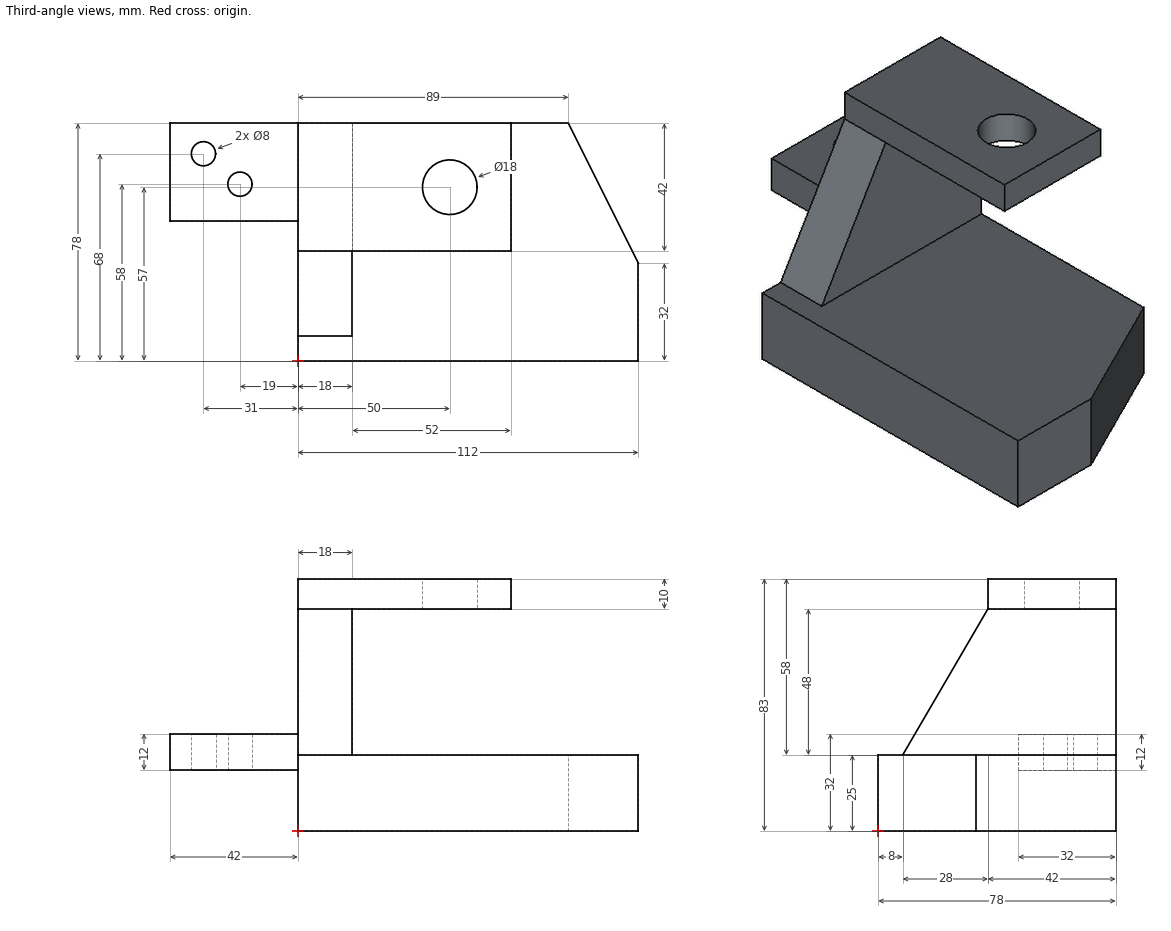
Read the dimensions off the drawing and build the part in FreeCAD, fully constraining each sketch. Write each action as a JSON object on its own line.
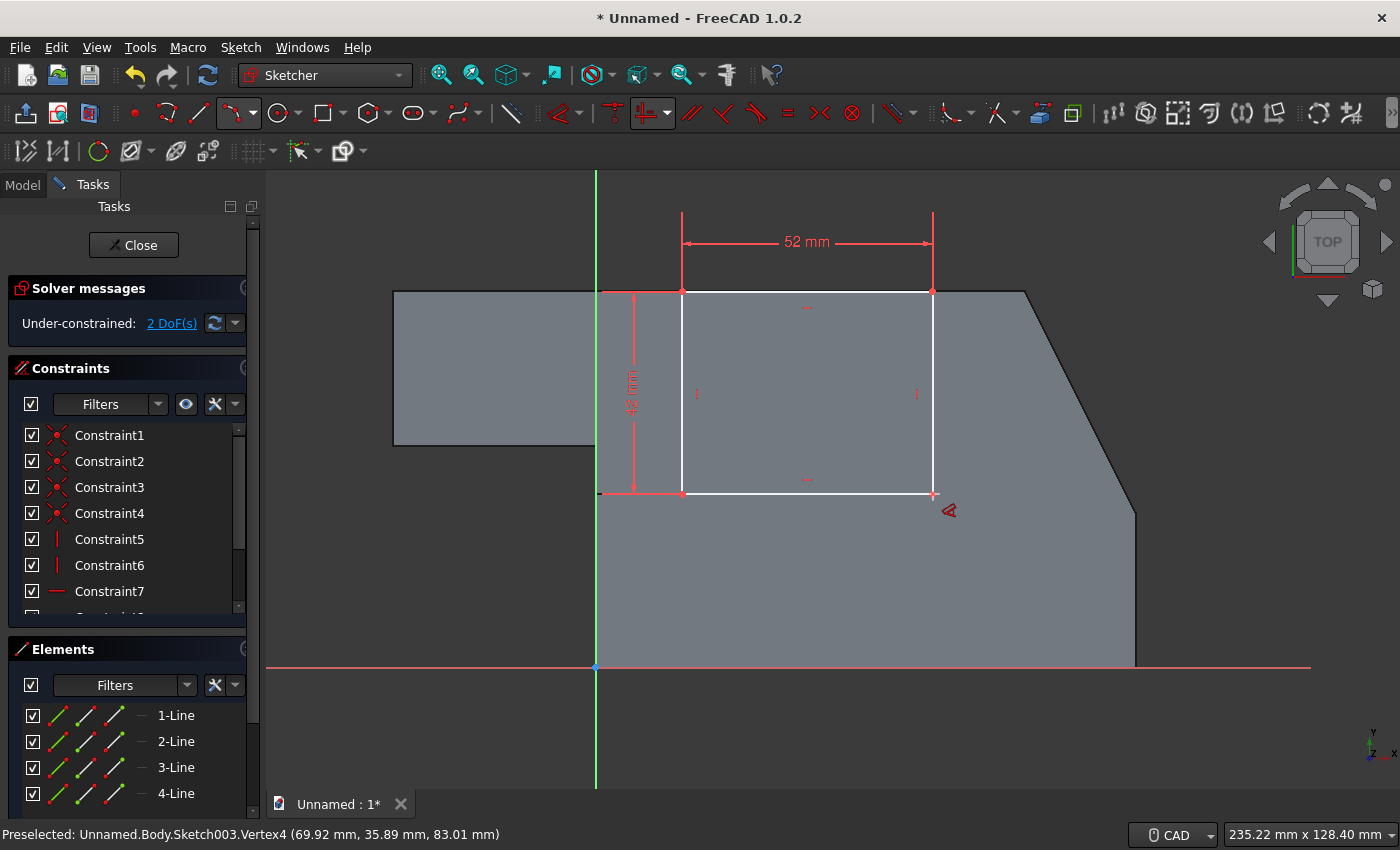
{"action": "left_click", "coordinate": [682, 292]}
{"action": "left_click", "coordinate": [639, 702]}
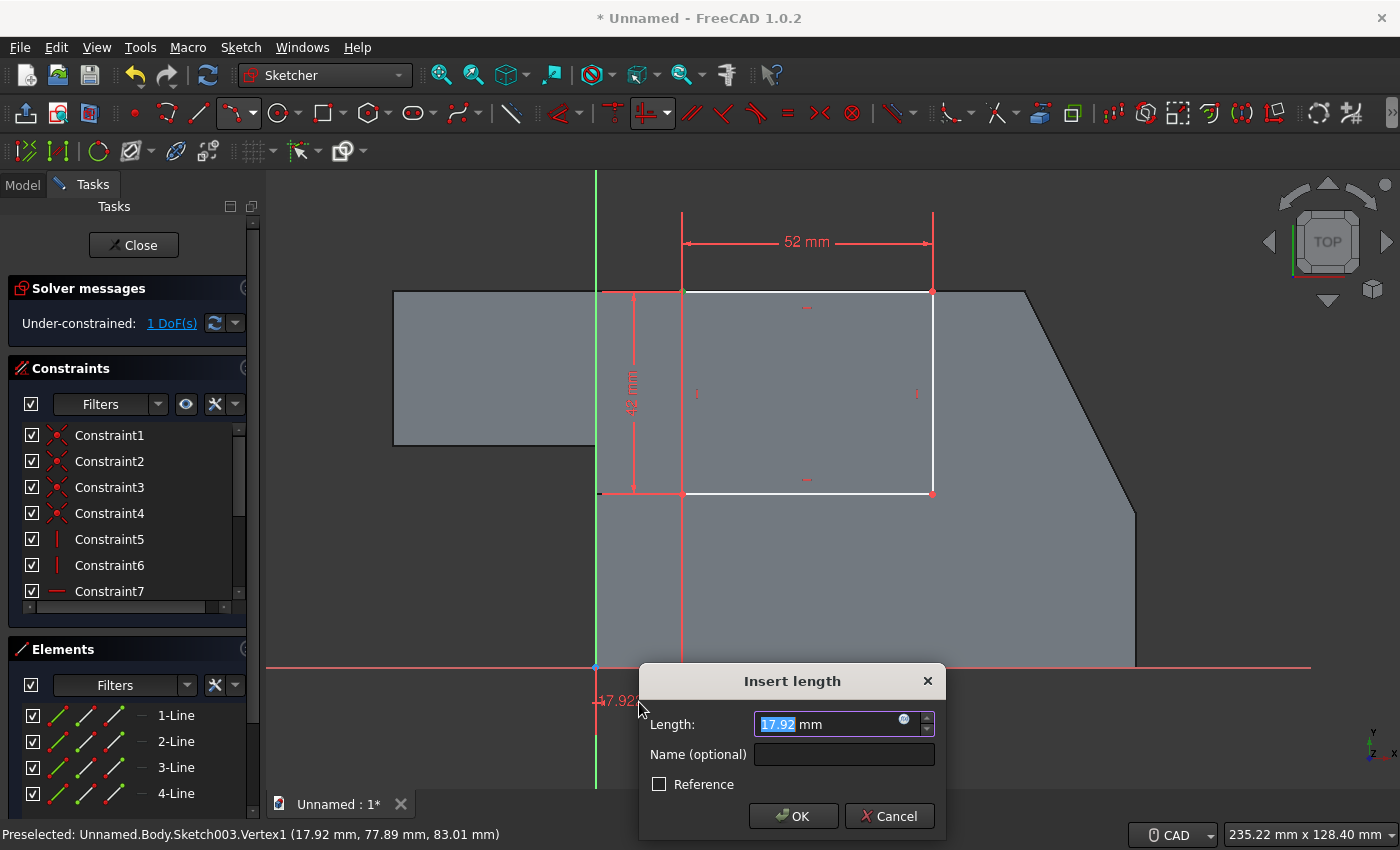
{"action": "type", "text": "18"}
{"action": "key", "text": "Return"}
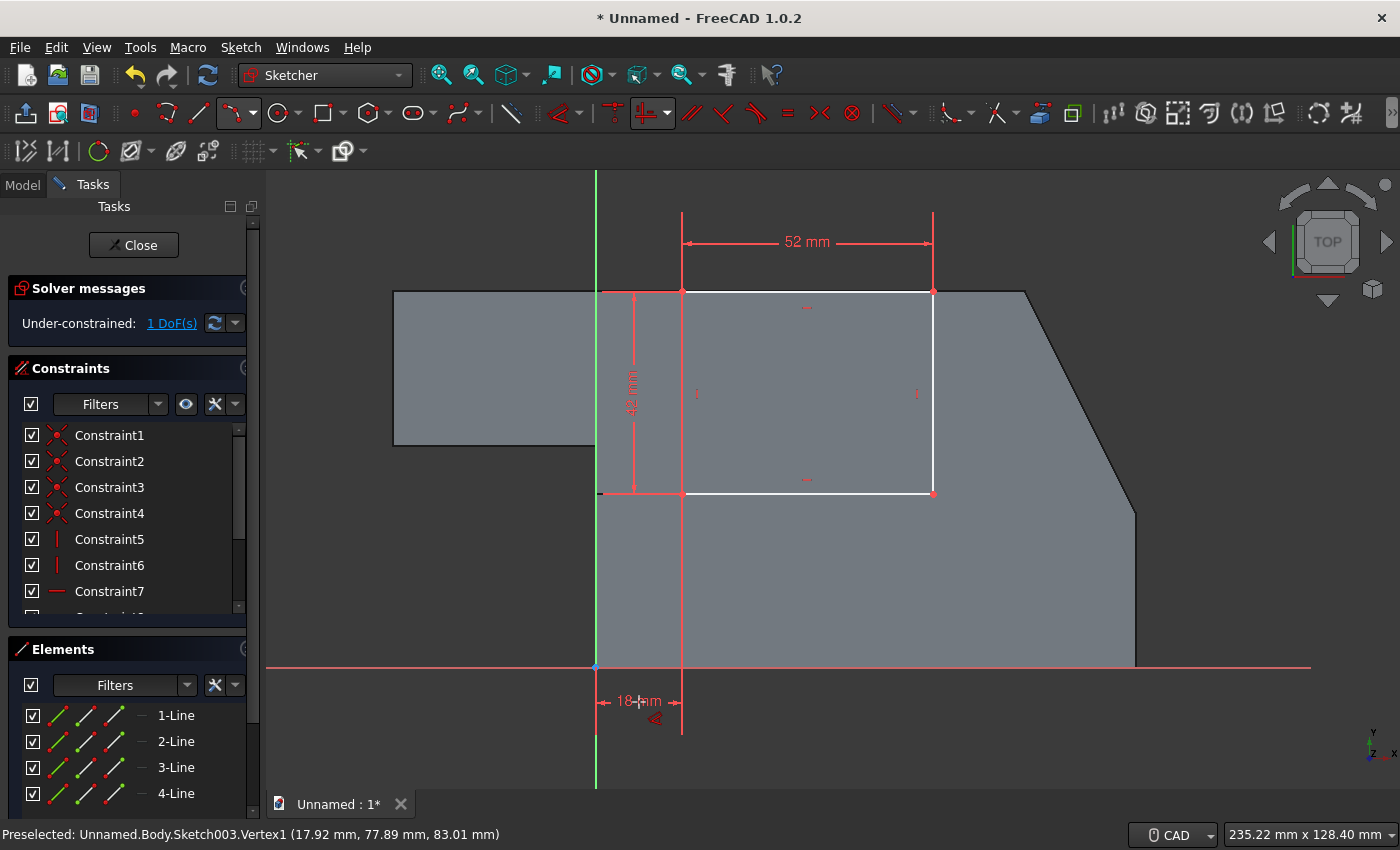
{"action": "left_click", "coordinate": [682, 292]}
{"action": "left_click", "coordinate": [562, 480]}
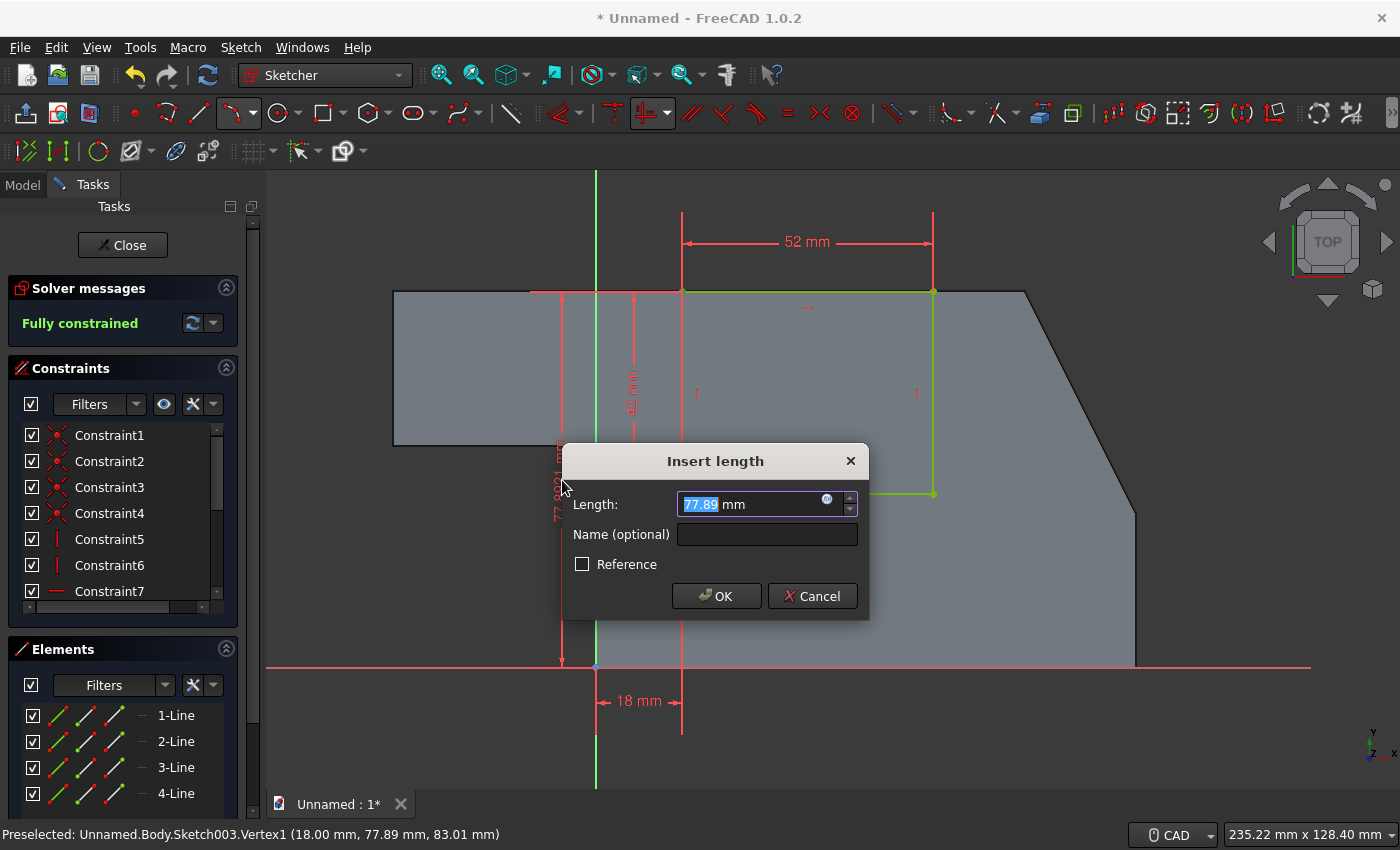
{"action": "type", "text": "78"}
{"action": "key", "text": "Return"}
{"action": "key", "text": "Escape"}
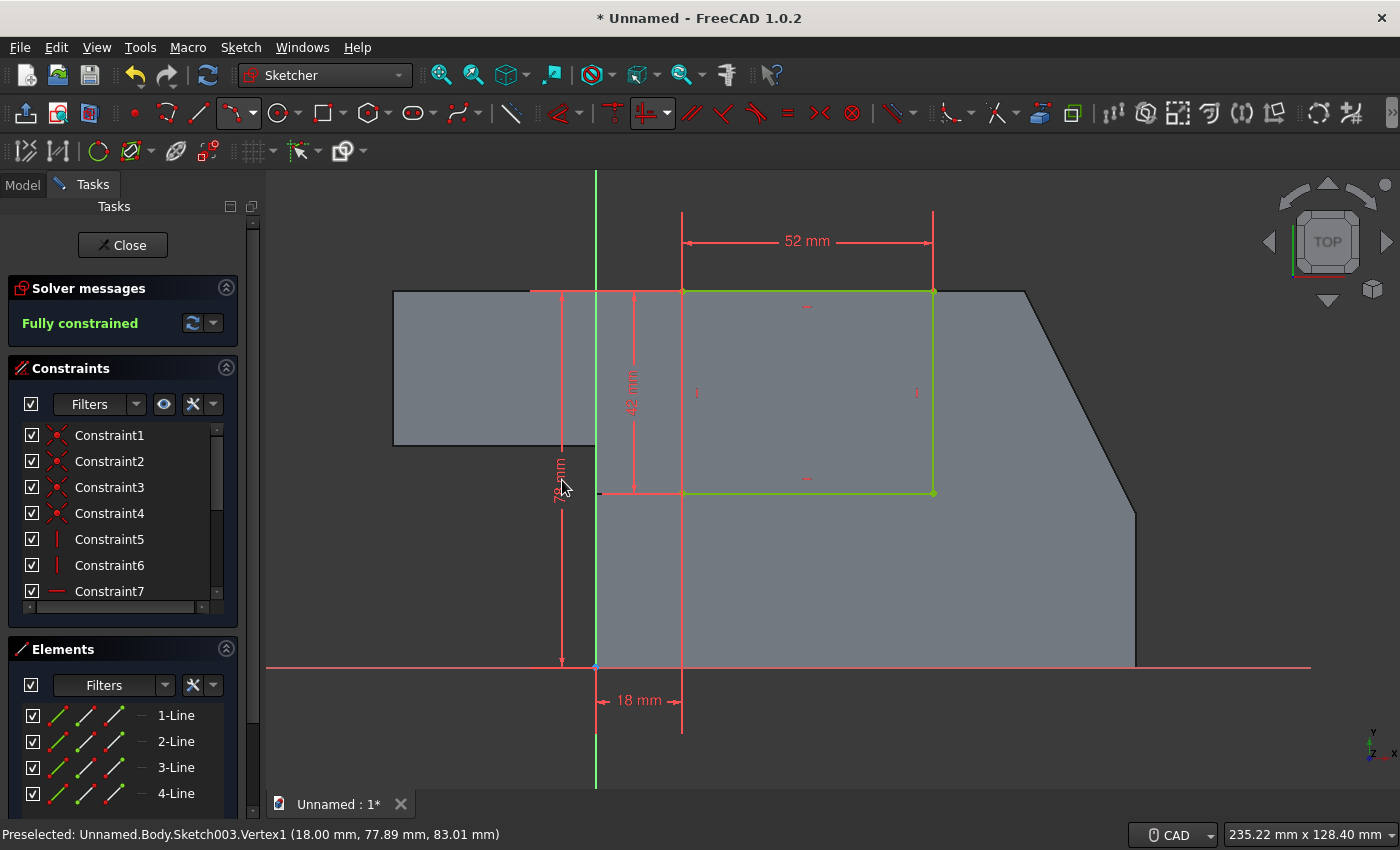
{"action": "left_click", "coordinate": [123, 245]}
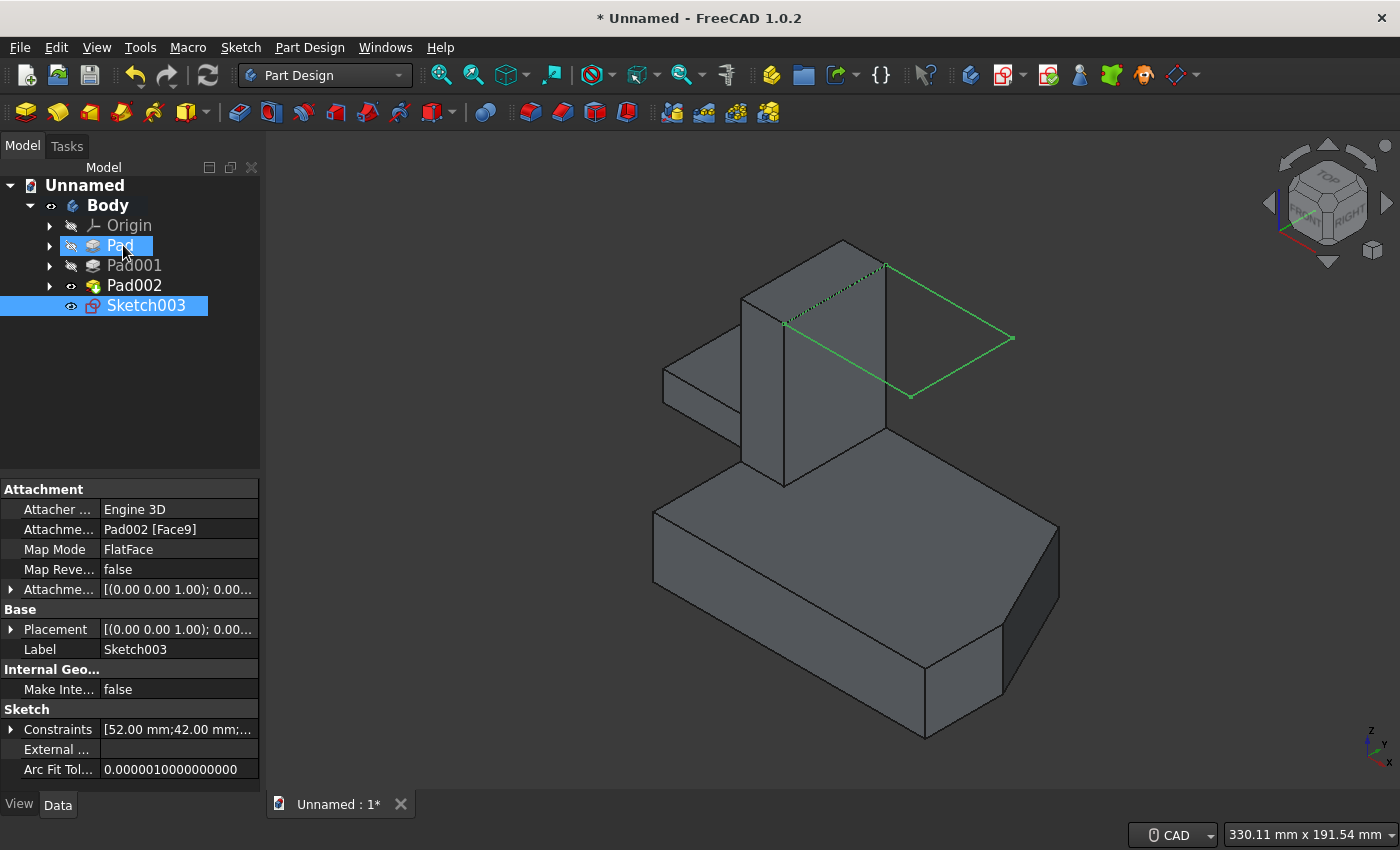
{"action": "left_click", "coordinate": [26, 112]}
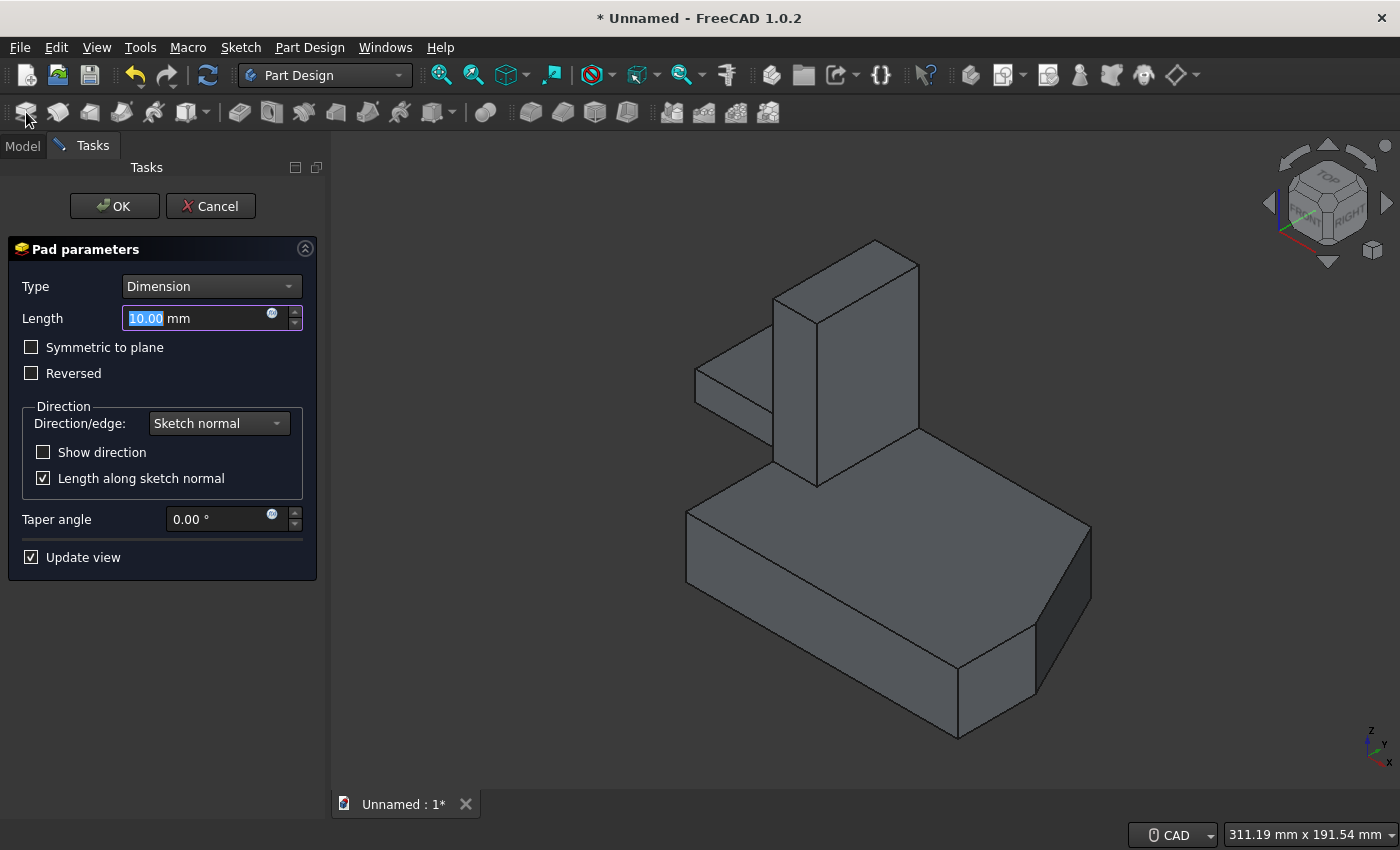
{"action": "type", "text": "10"}
{"action": "key", "text": "Tab"}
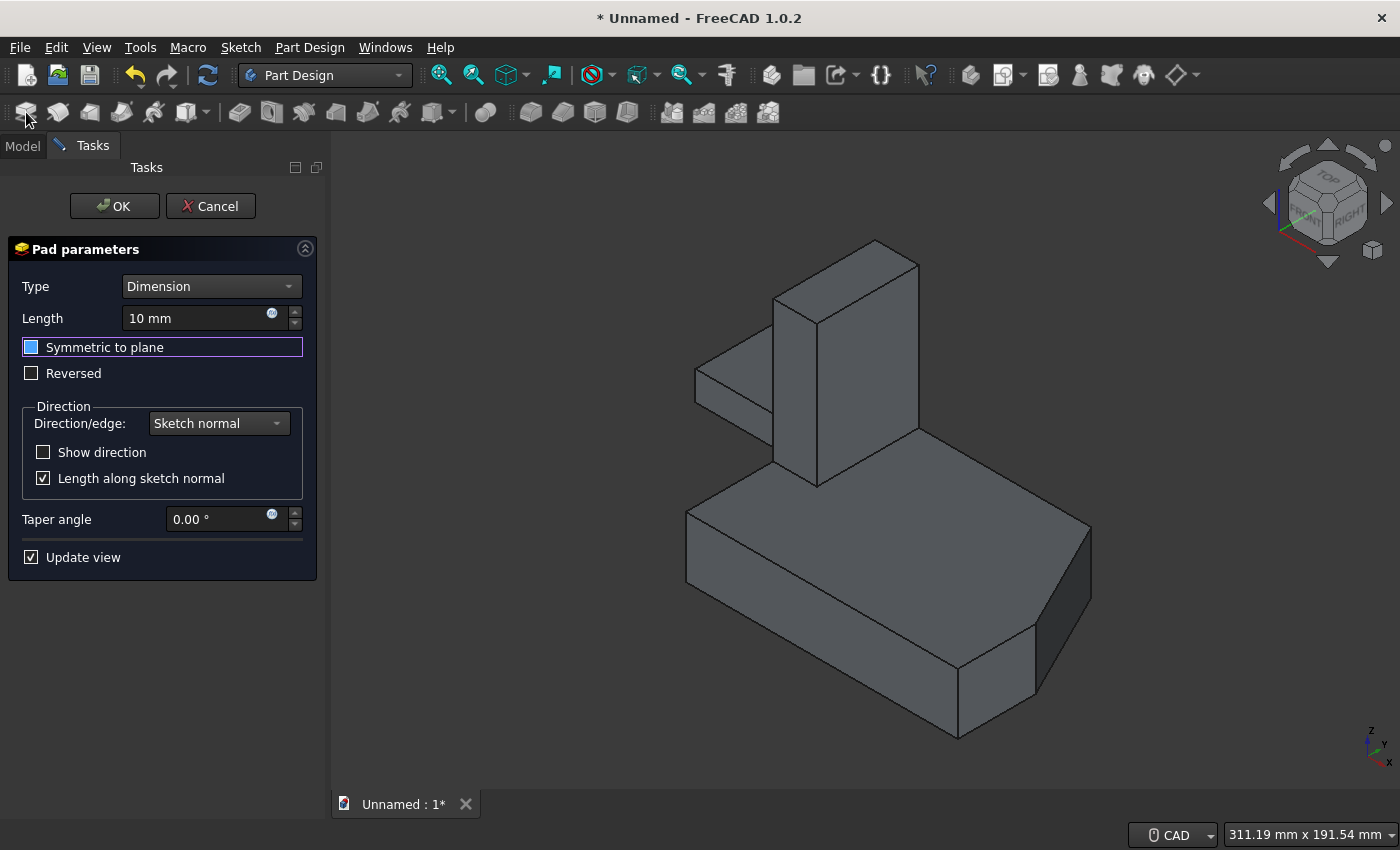
{"action": "left_click", "coordinate": [30, 373]}